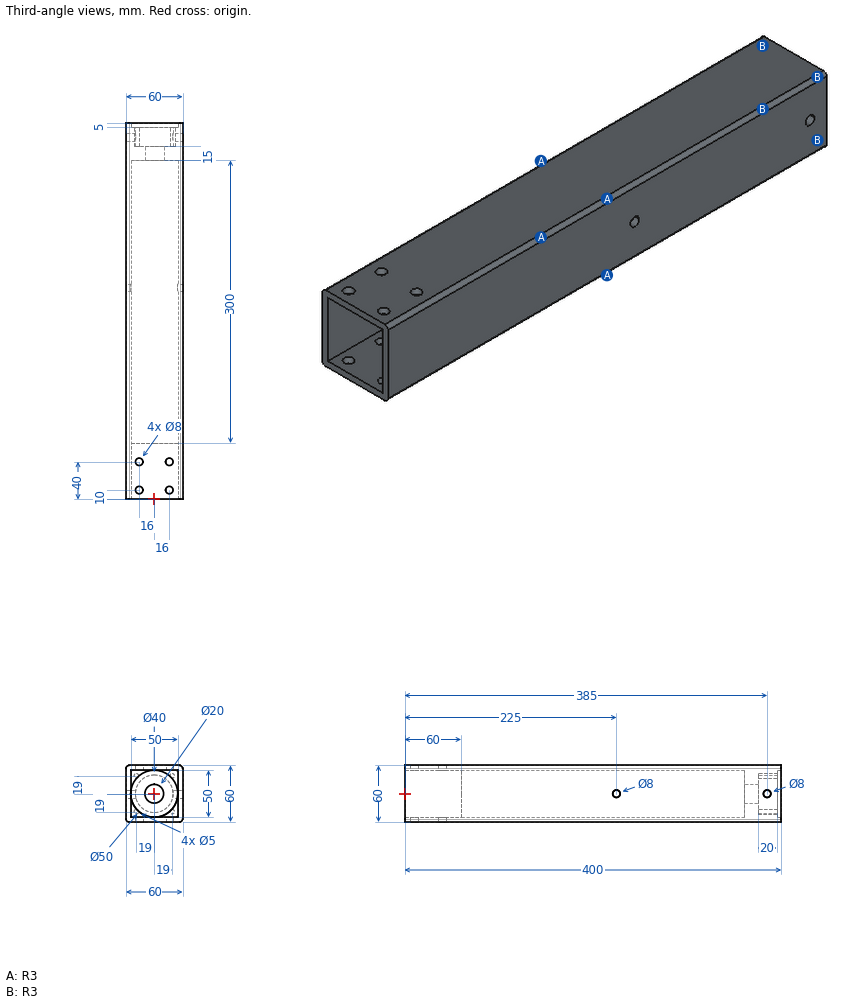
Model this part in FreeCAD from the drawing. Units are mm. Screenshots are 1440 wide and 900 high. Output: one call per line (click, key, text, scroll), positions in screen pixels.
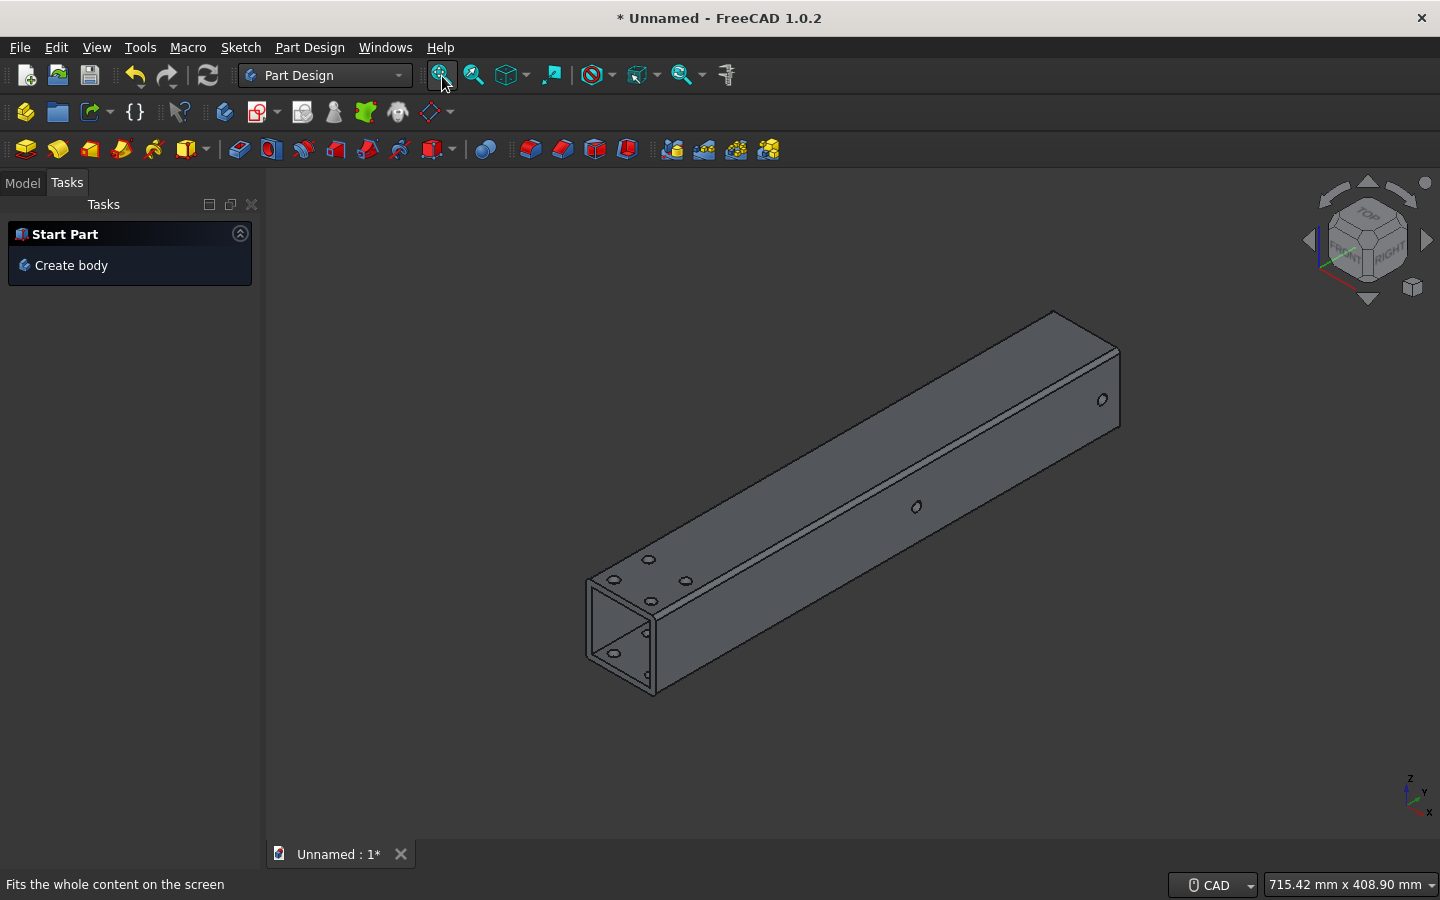
key(2)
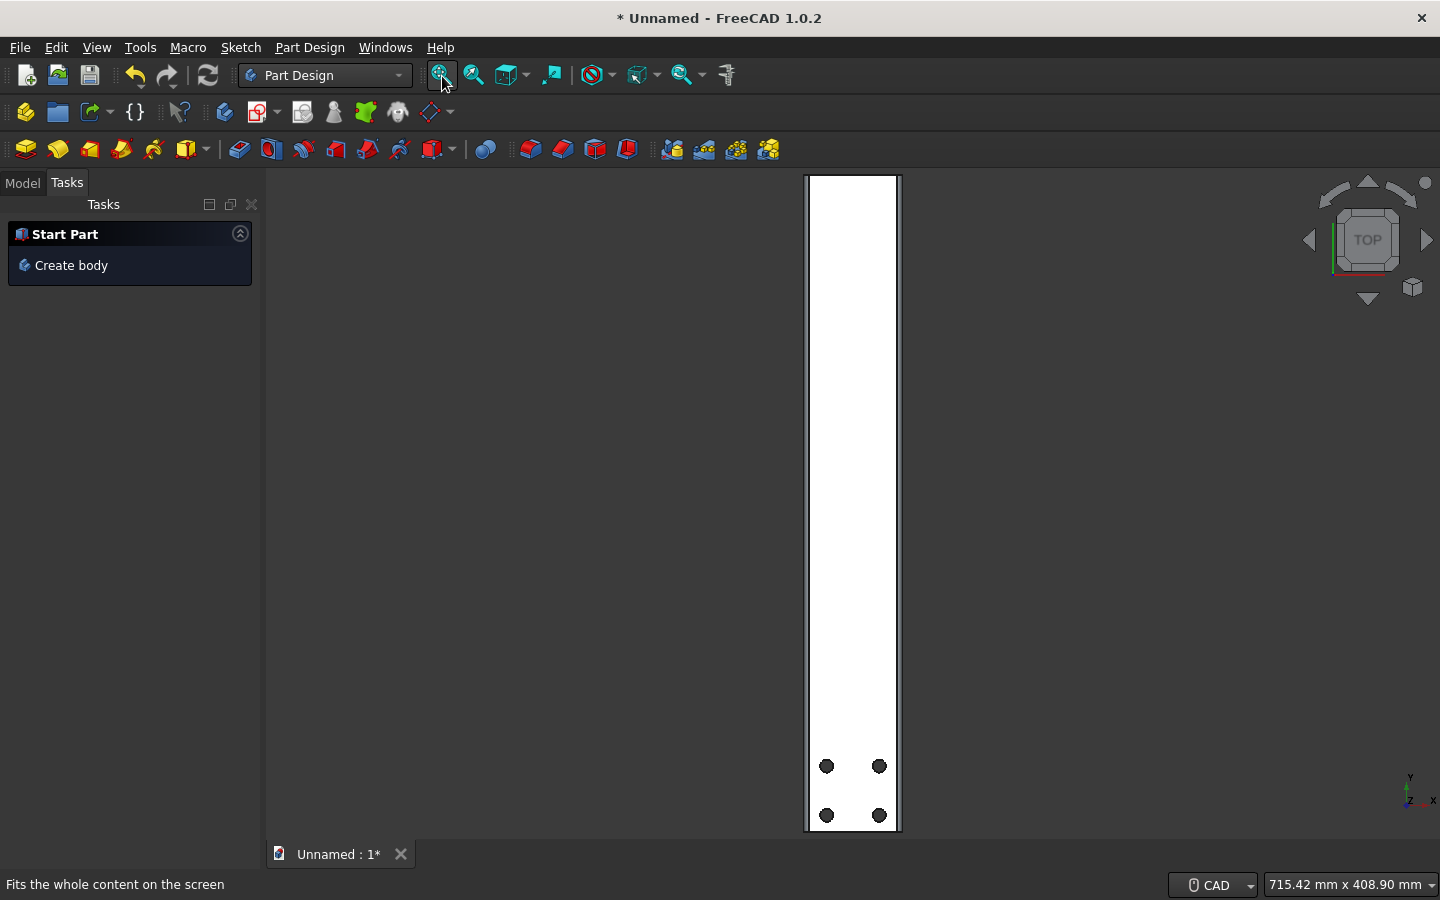
key(1)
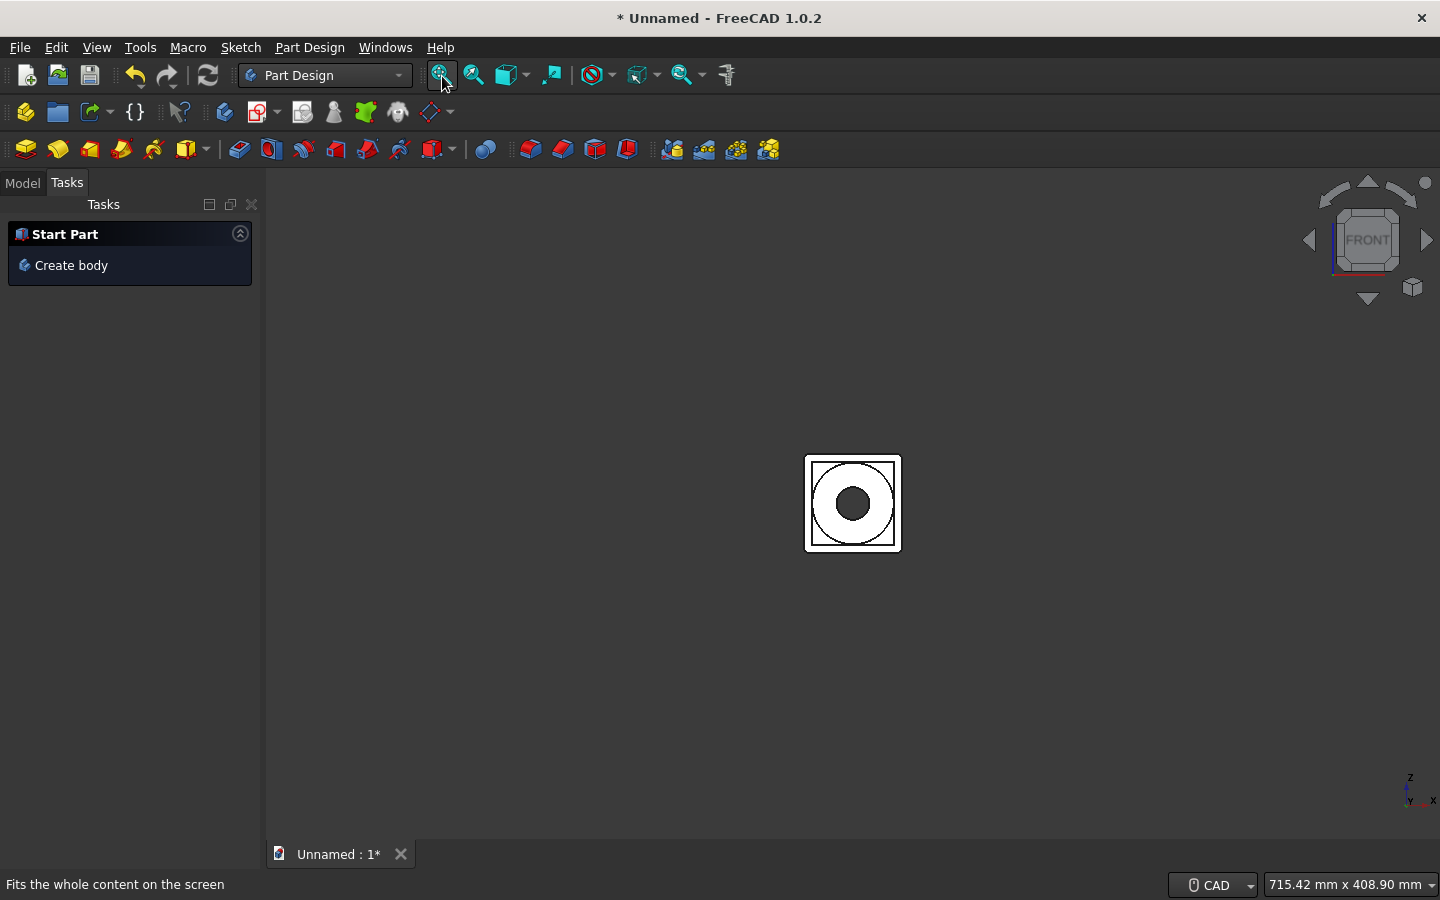
click(442, 76)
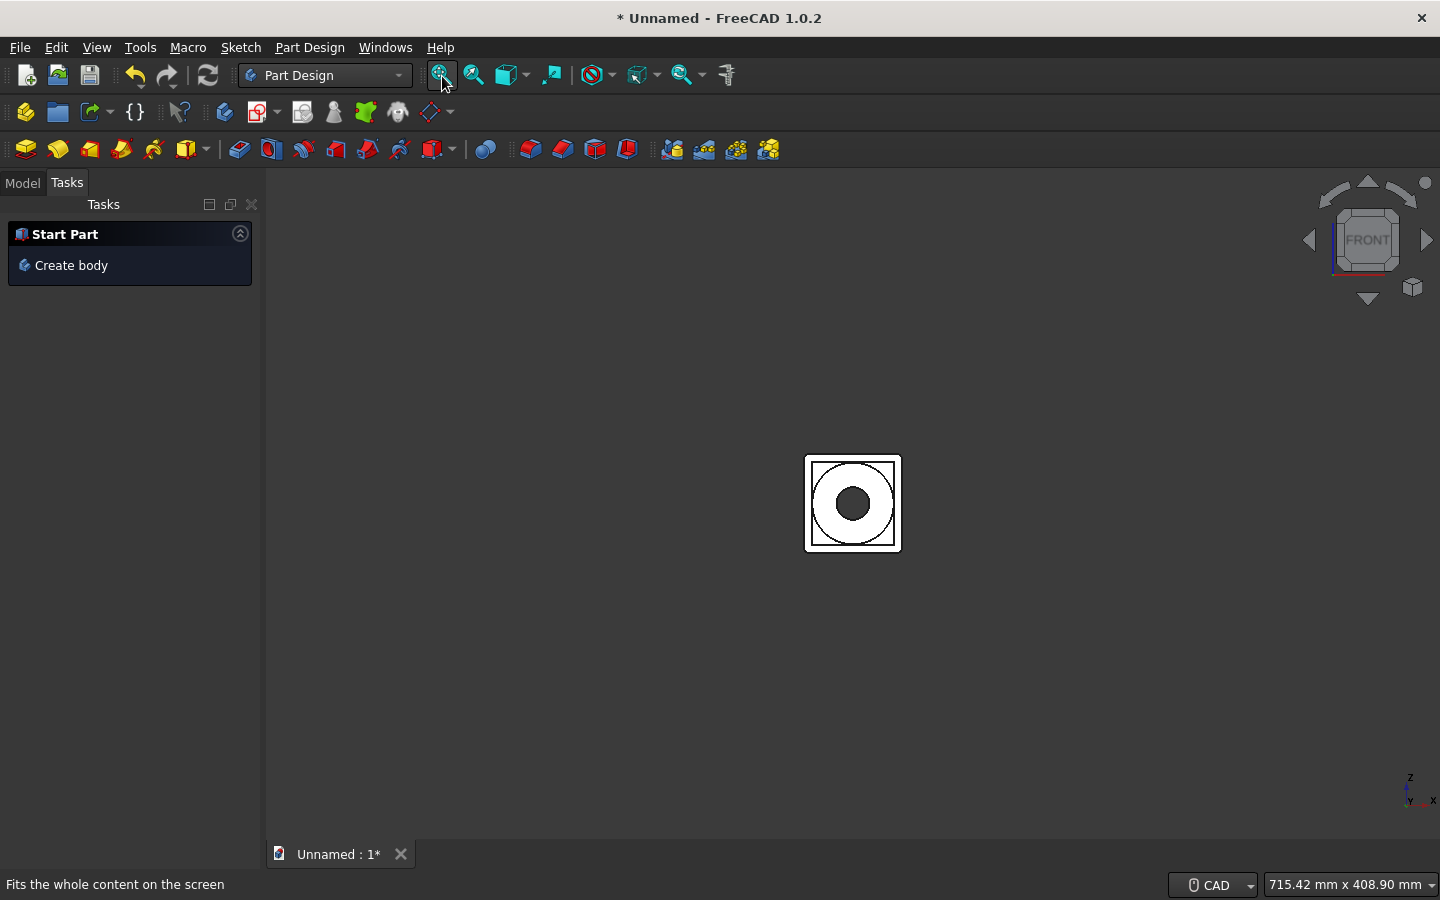
scroll(894, 544, up, 8)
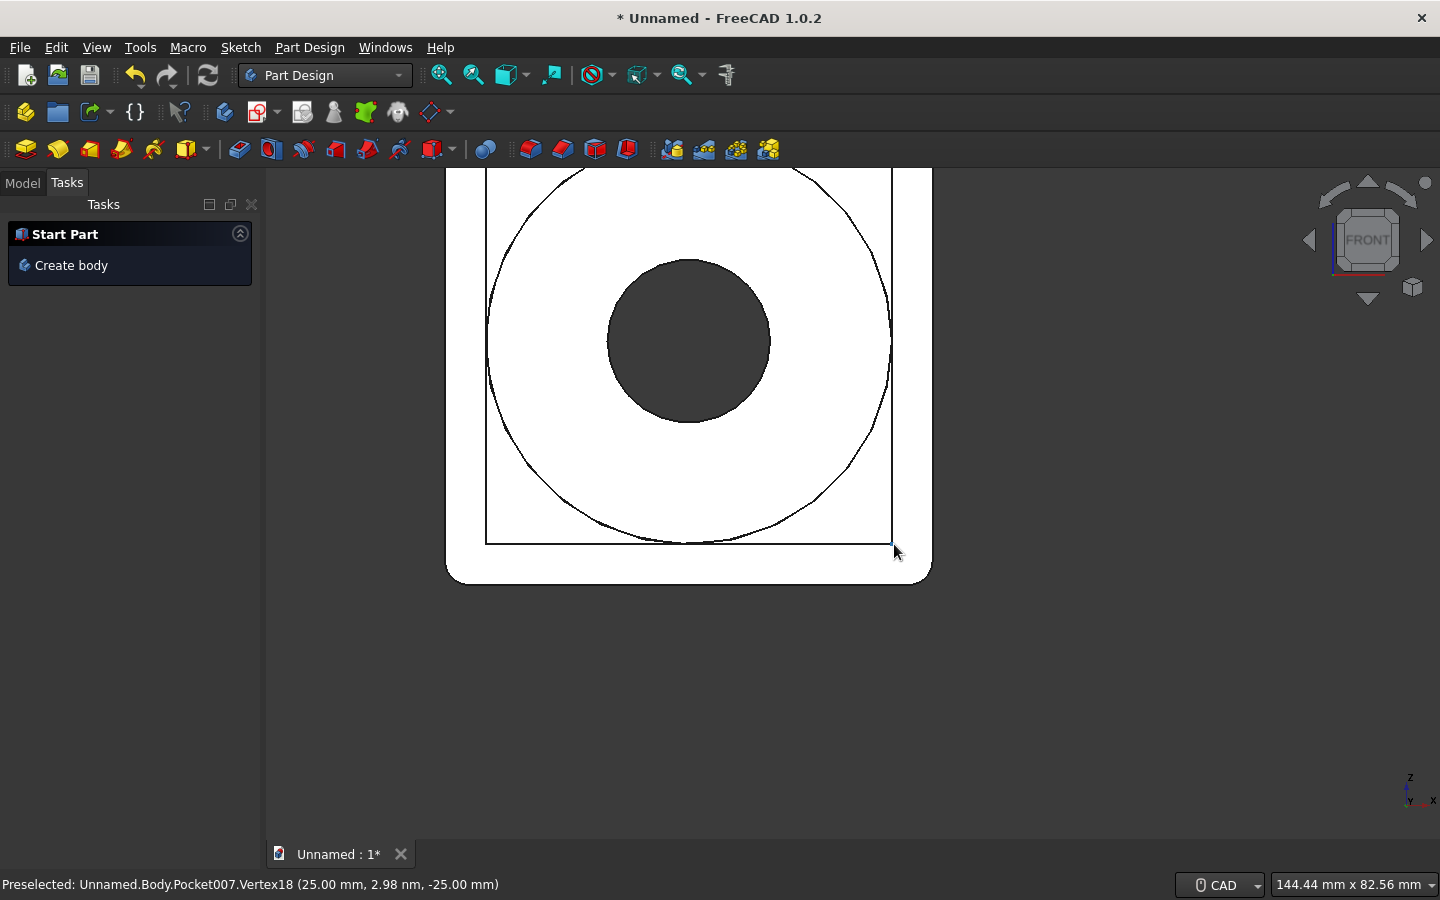
click(442, 76)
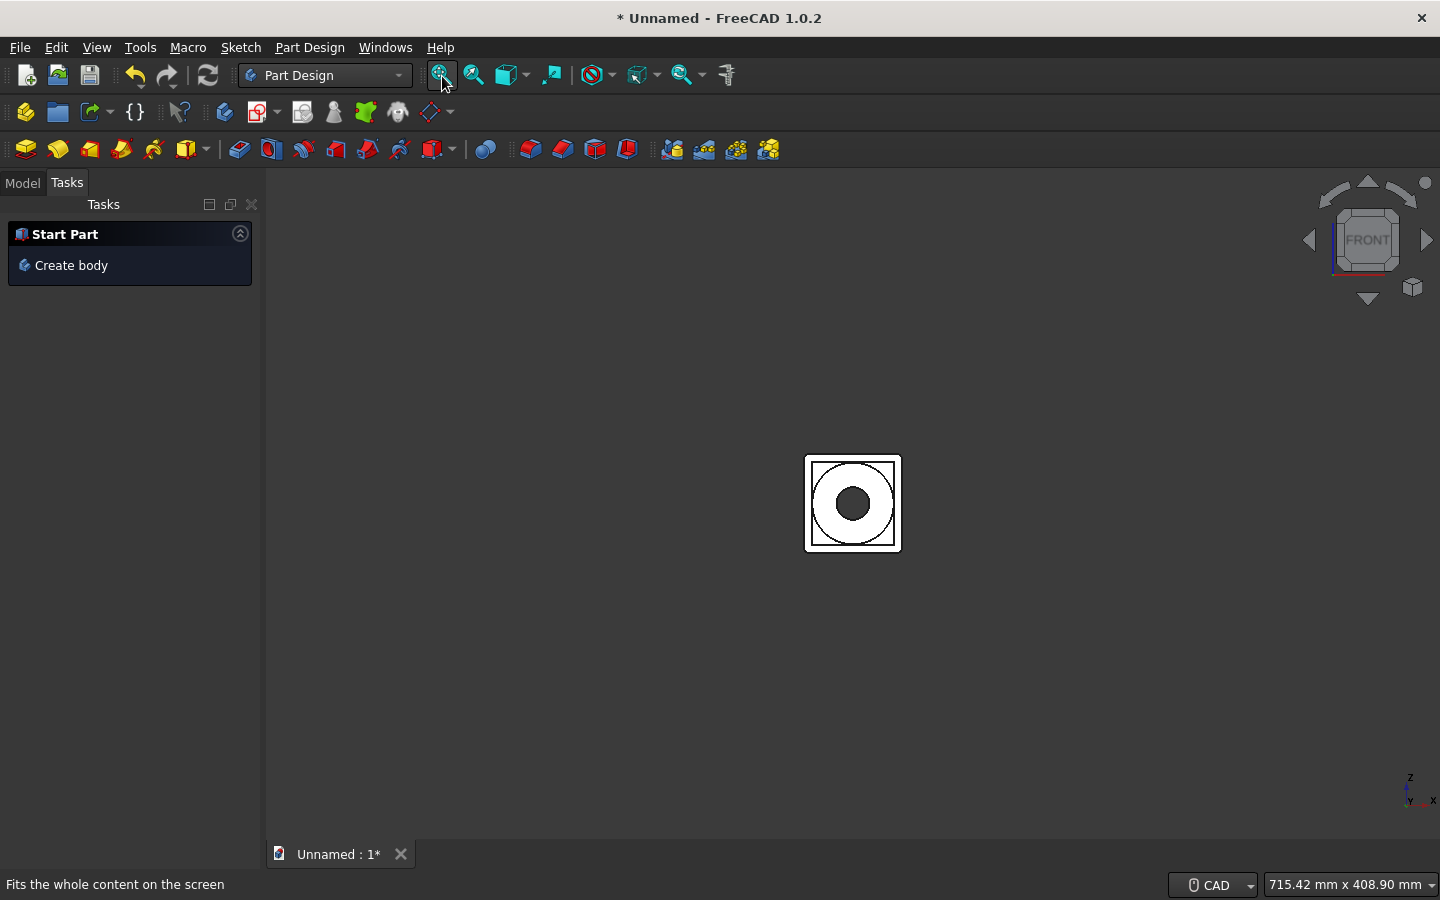
key(3)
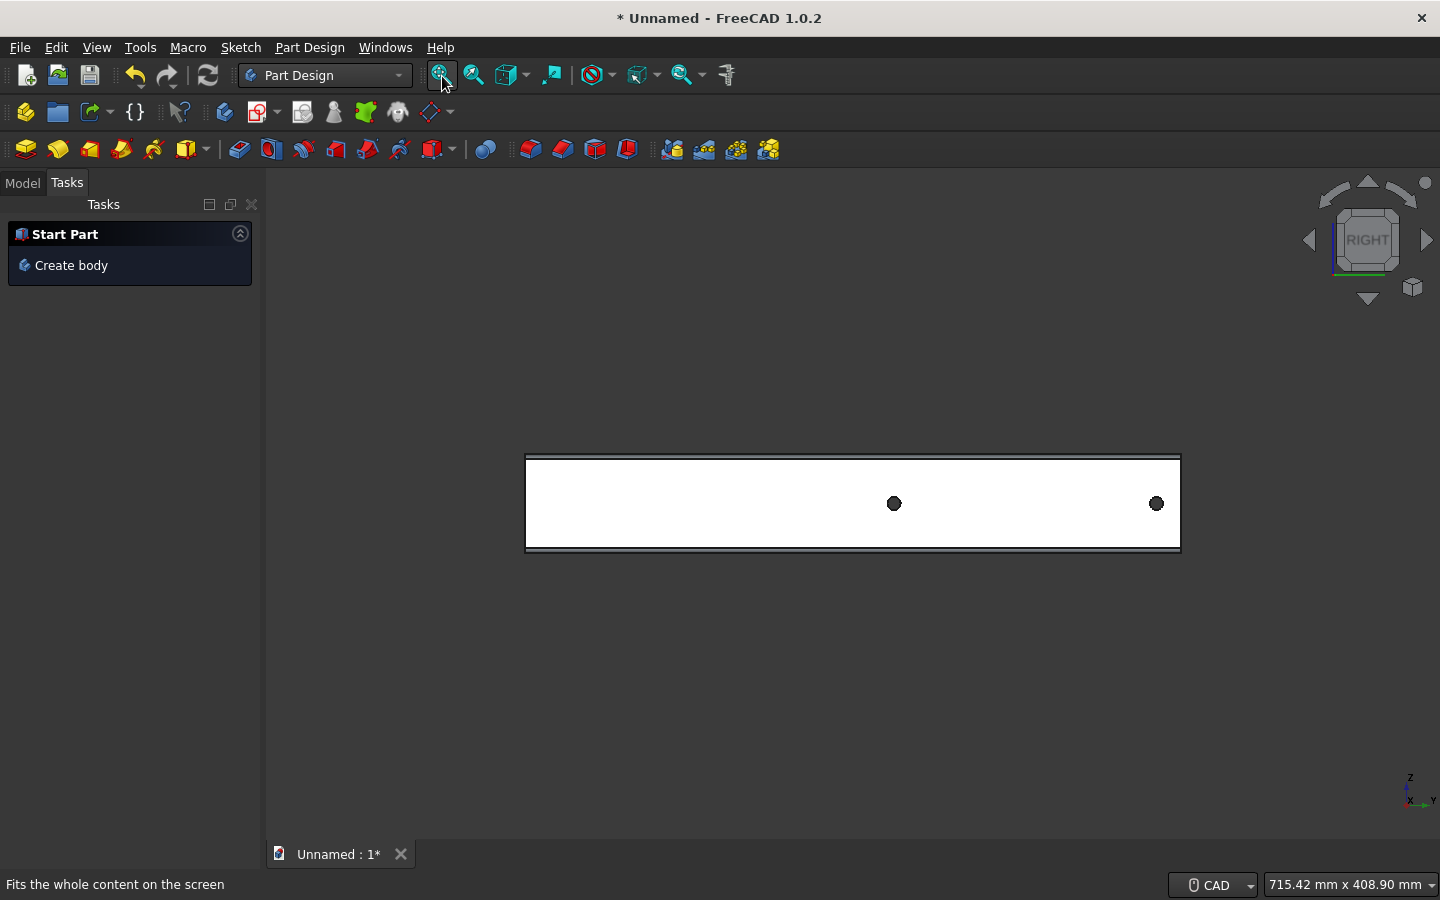
scroll(1177, 544, up, 8)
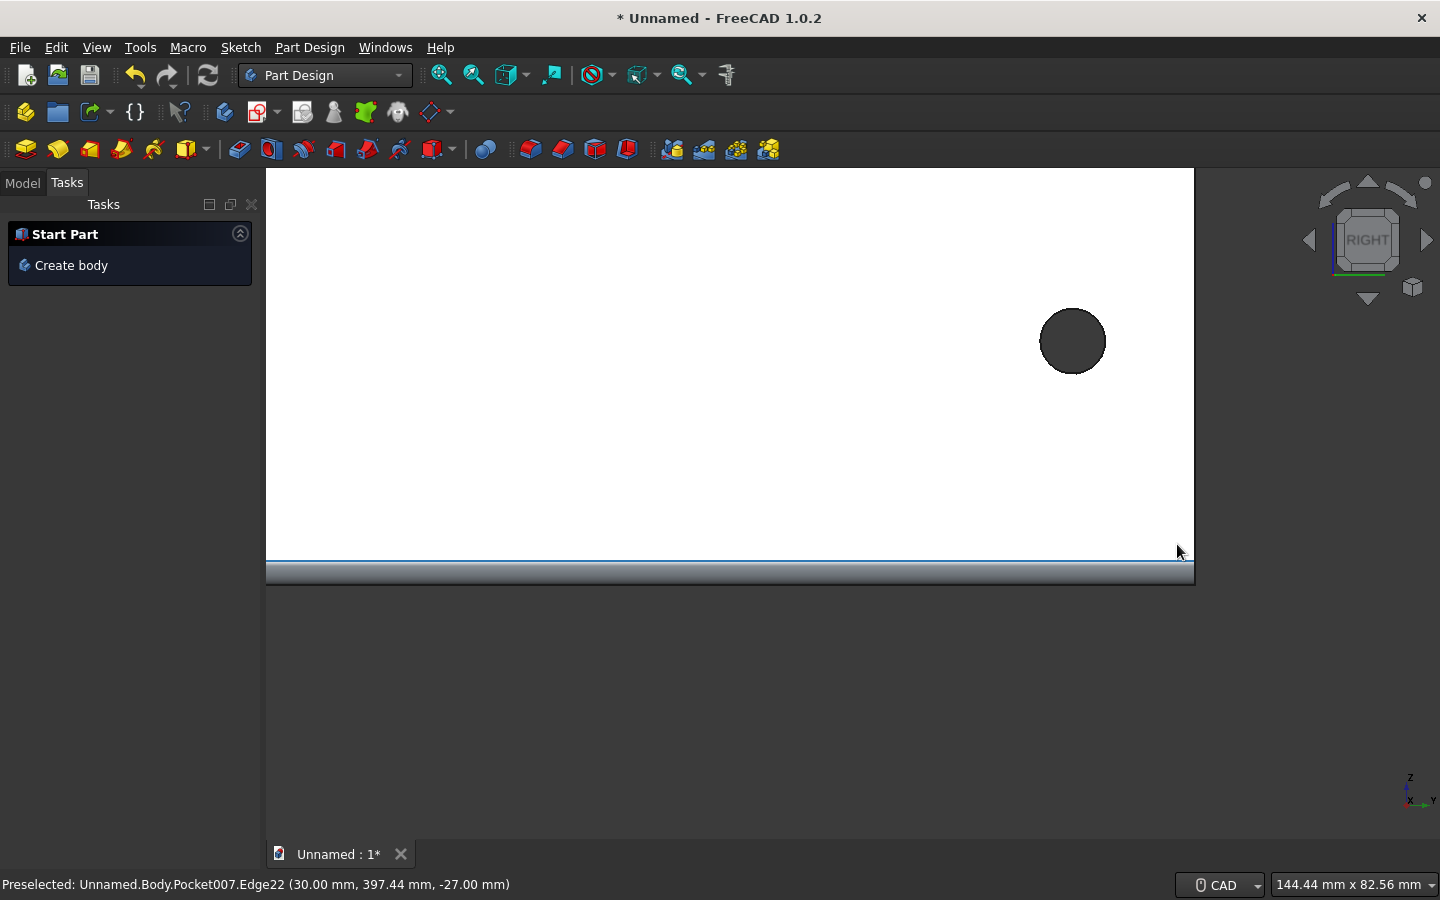
click(442, 76)